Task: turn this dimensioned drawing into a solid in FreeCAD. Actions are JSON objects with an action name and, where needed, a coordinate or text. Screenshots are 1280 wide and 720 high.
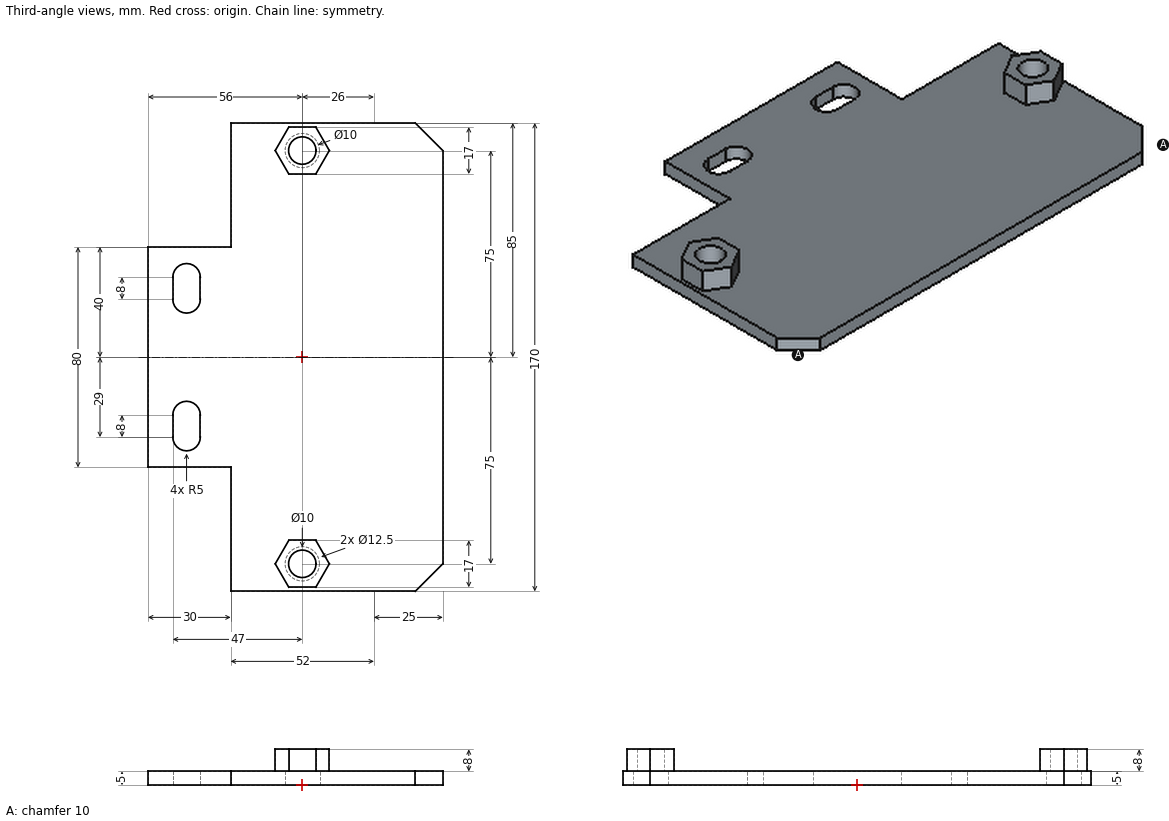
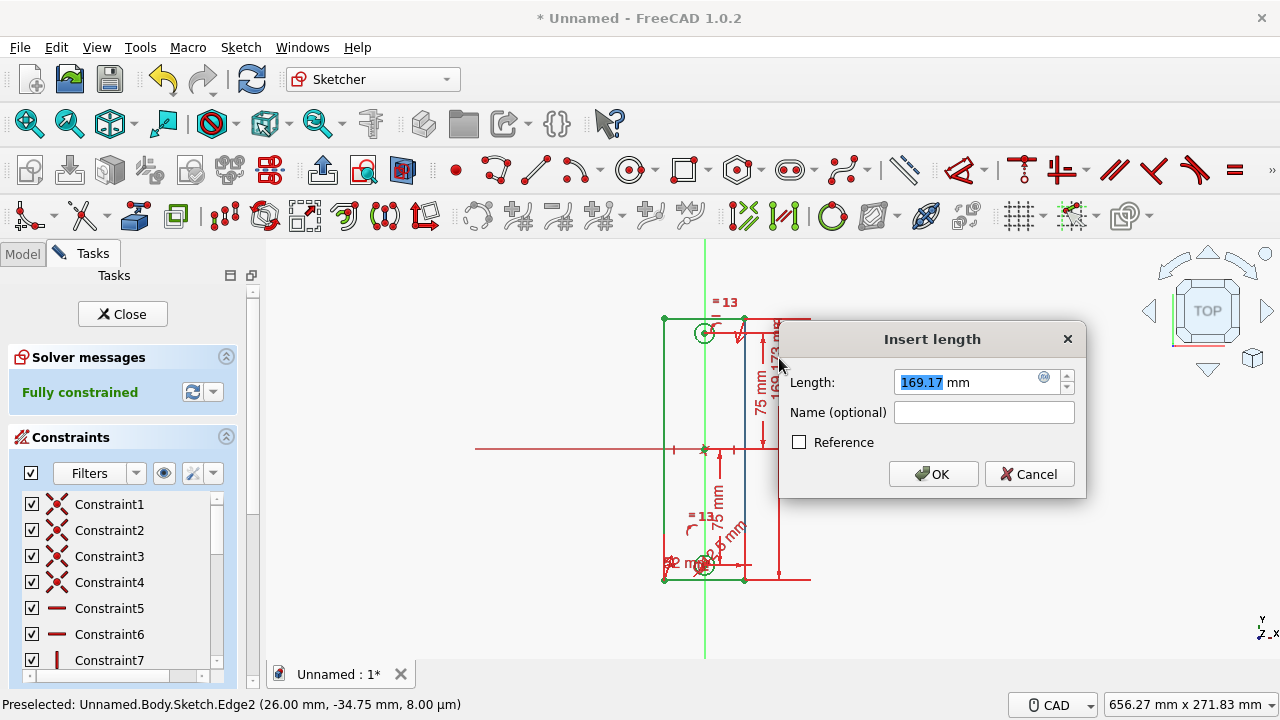
{"action": "type", "text": "170"}
{"action": "key", "text": "Return"}
{"action": "key", "text": "Escape"}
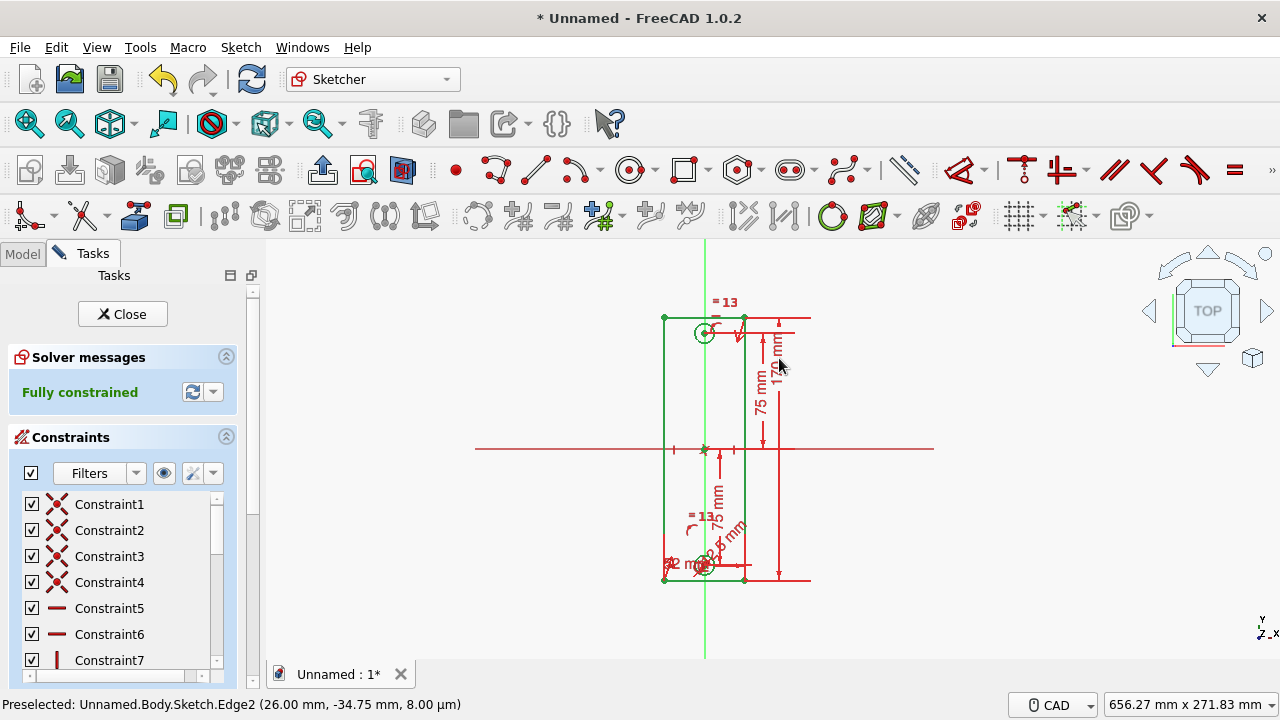
{"action": "left_click", "coordinate": [123, 314]}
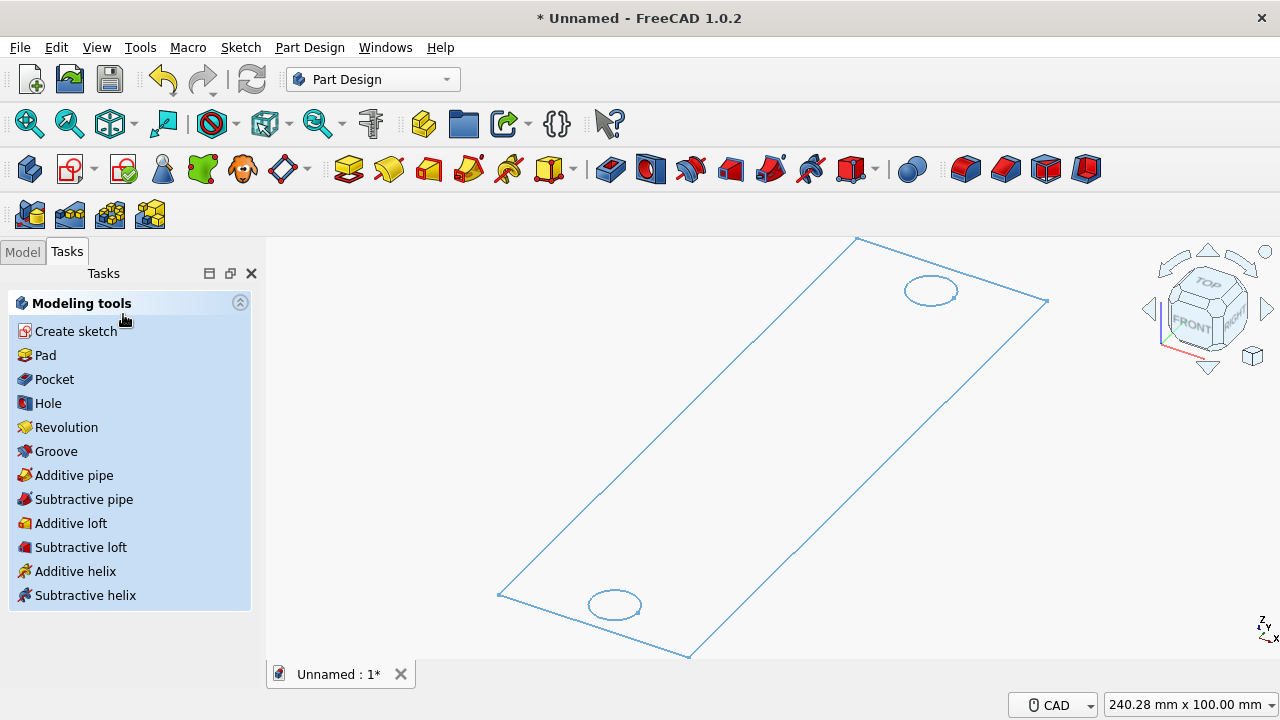
{"action": "left_click", "coordinate": [350, 170]}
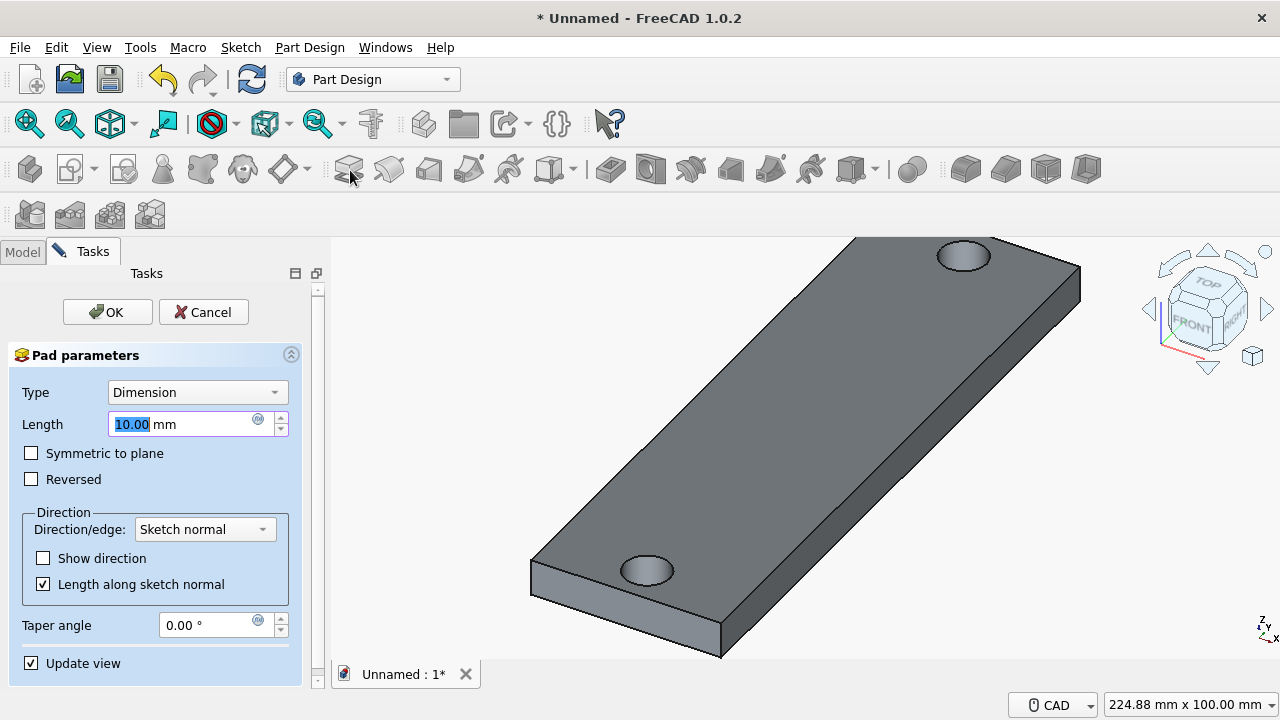
{"action": "type", "text": "5"}
{"action": "key", "text": "Tab"}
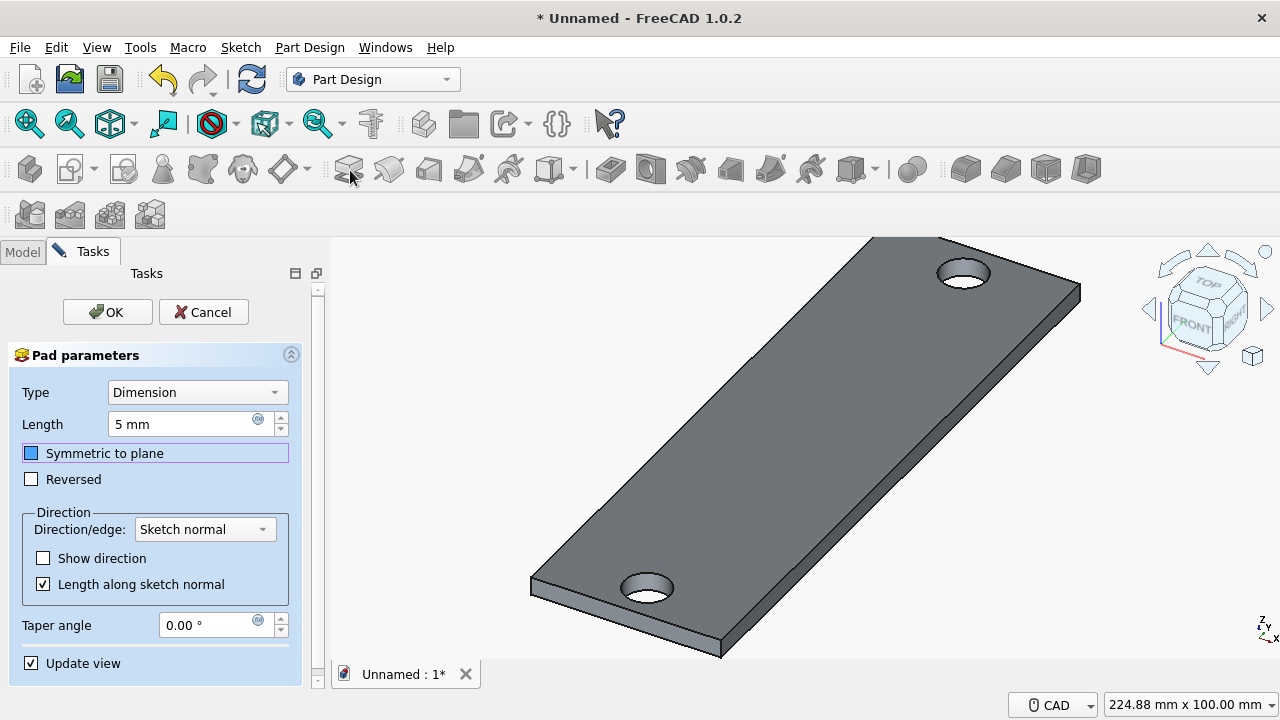
{"action": "left_click", "coordinate": [108, 312]}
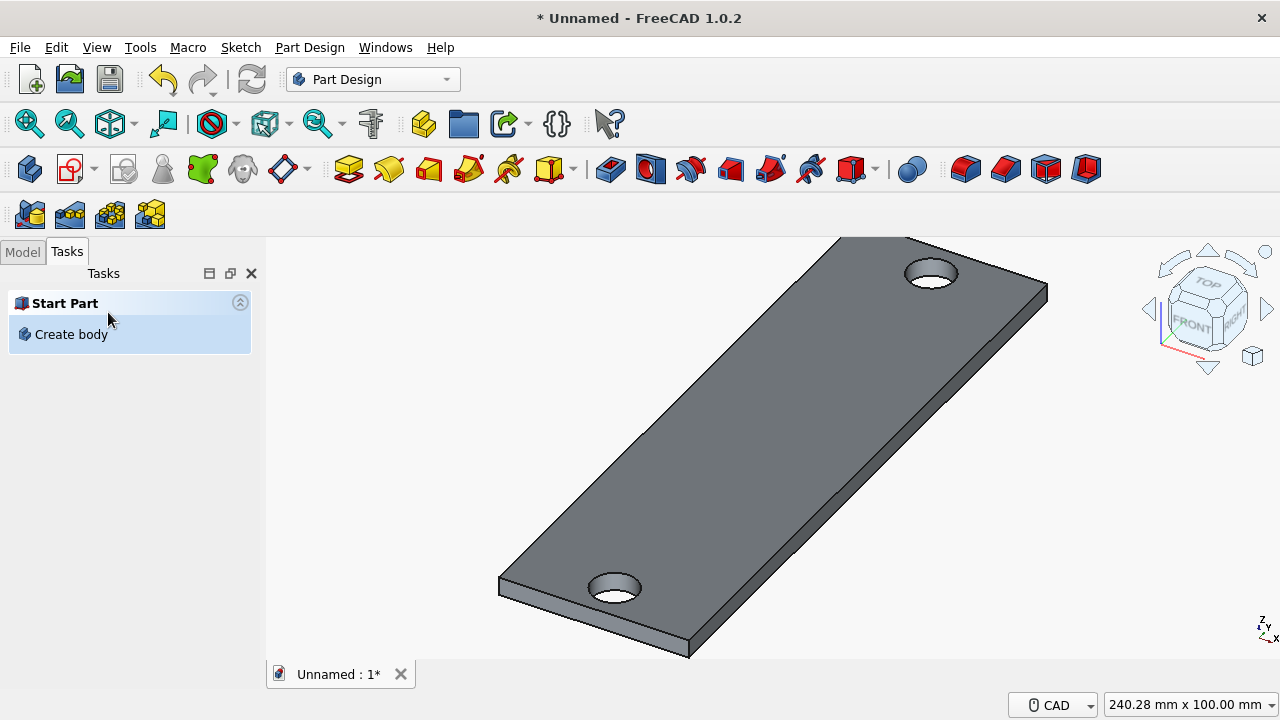
{"action": "left_click", "coordinate": [30, 124]}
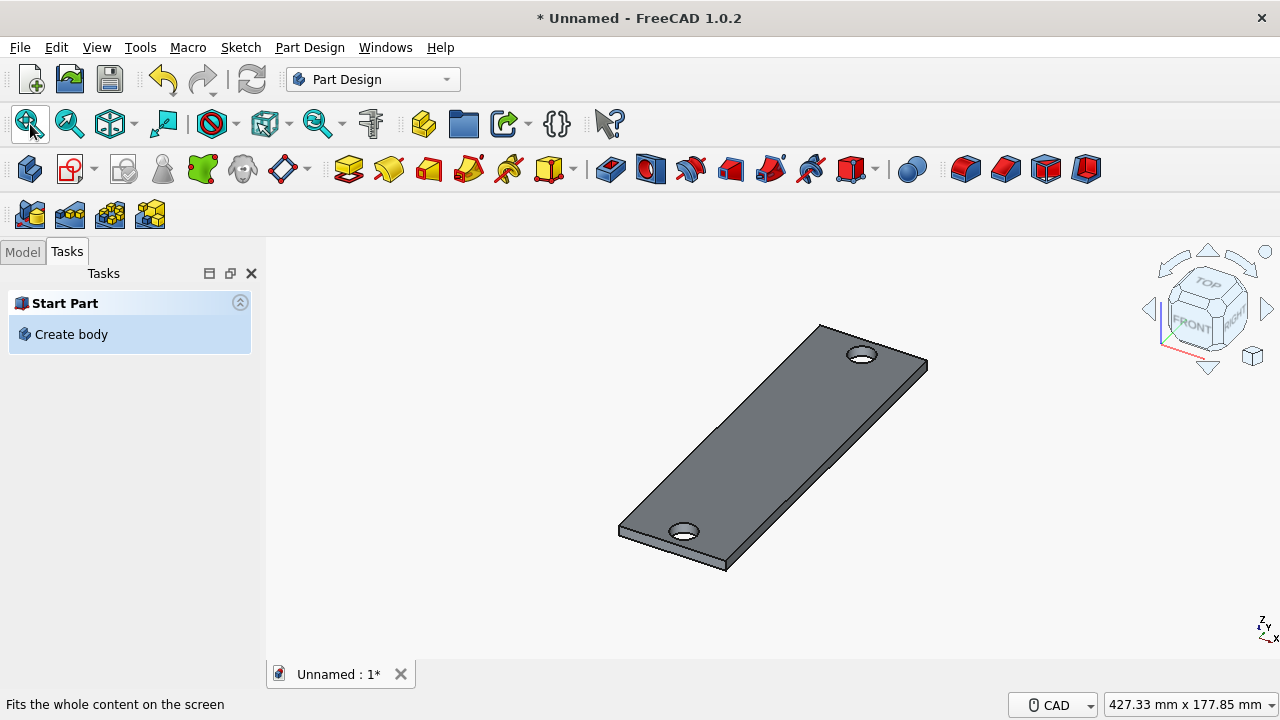
{"action": "left_click", "coordinate": [70, 170]}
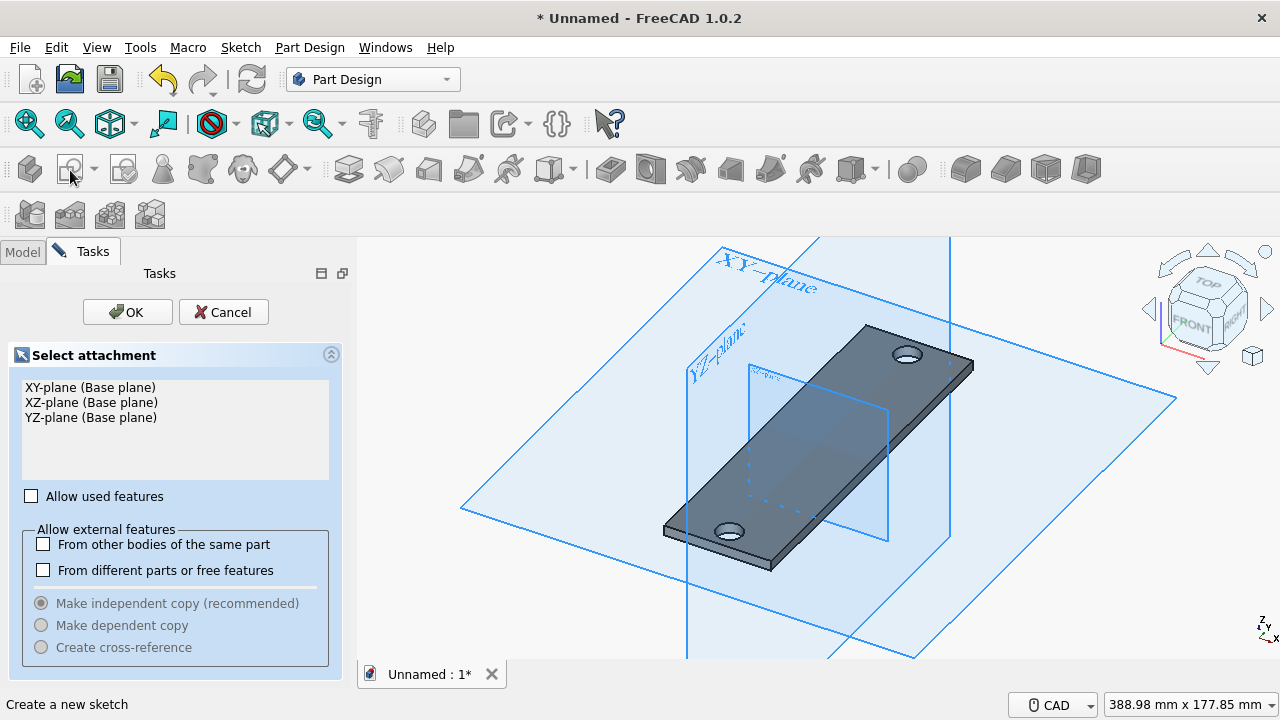
{"action": "left_click", "coordinate": [82, 388]}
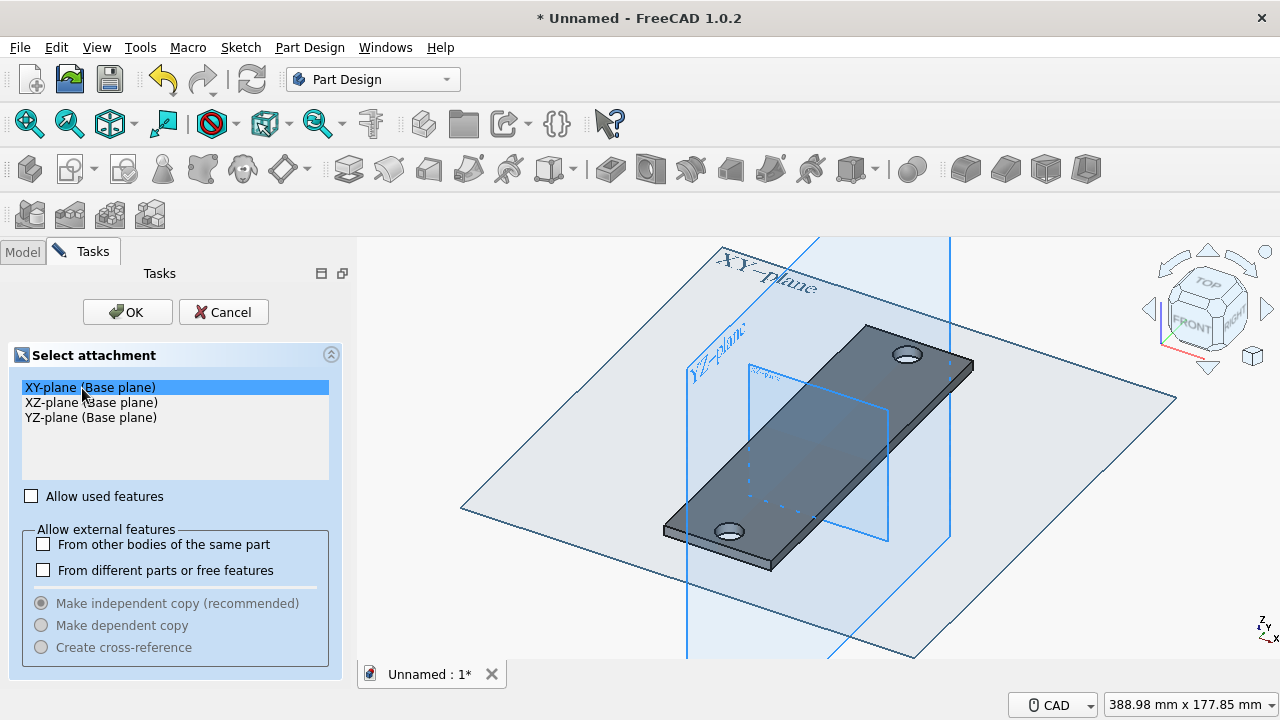
{"action": "left_click", "coordinate": [128, 312]}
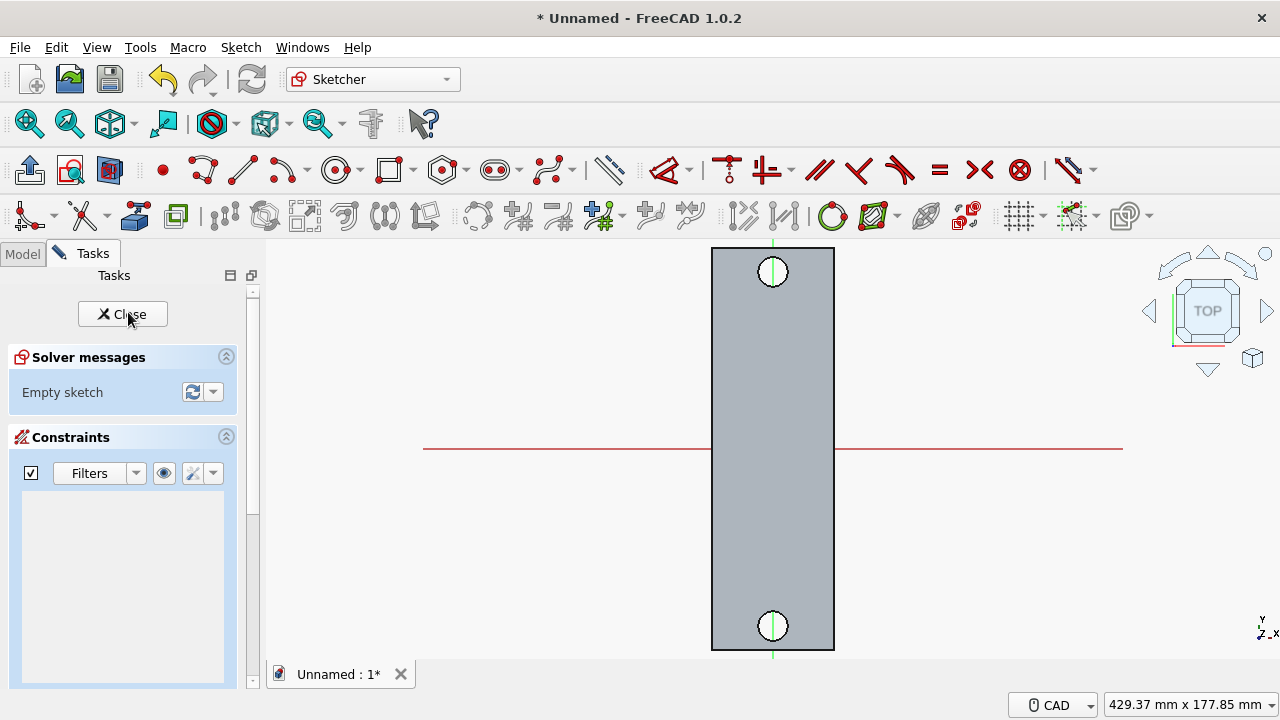
{"action": "left_click", "coordinate": [110, 170]}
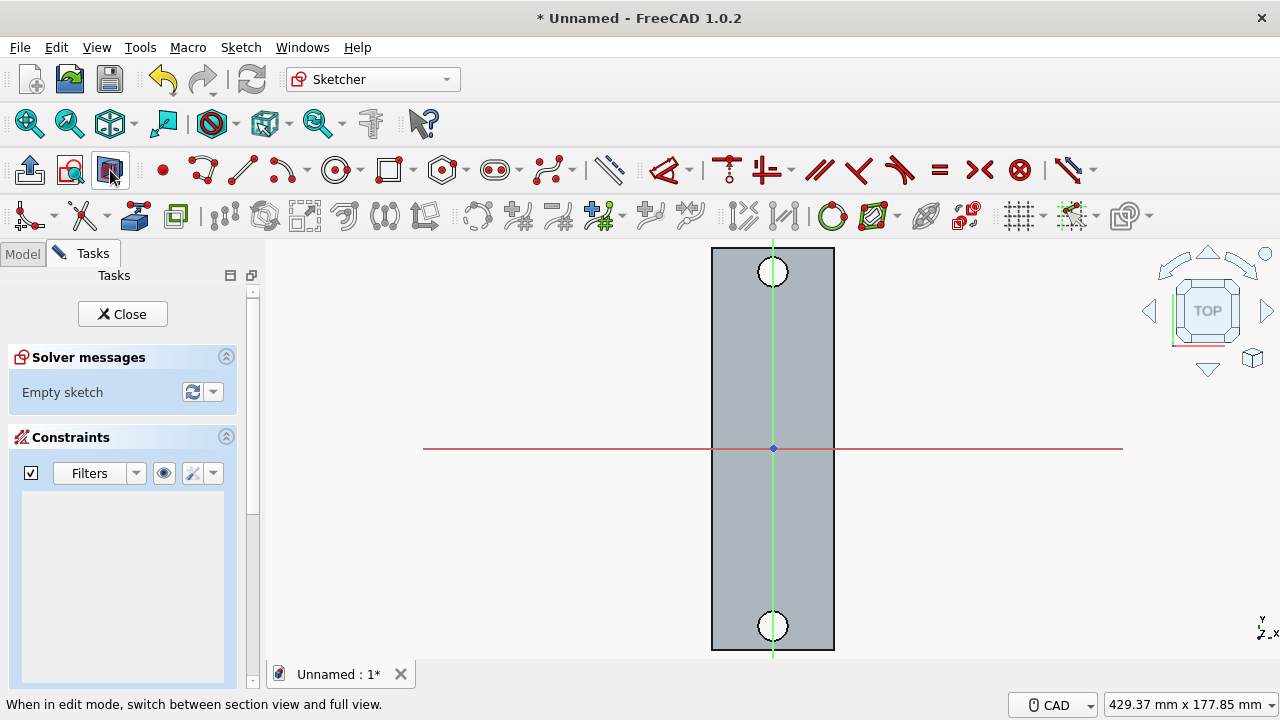
{"action": "scroll", "coordinate": [712, 449], "scroll_direction": "up", "scroll_amount": 2}